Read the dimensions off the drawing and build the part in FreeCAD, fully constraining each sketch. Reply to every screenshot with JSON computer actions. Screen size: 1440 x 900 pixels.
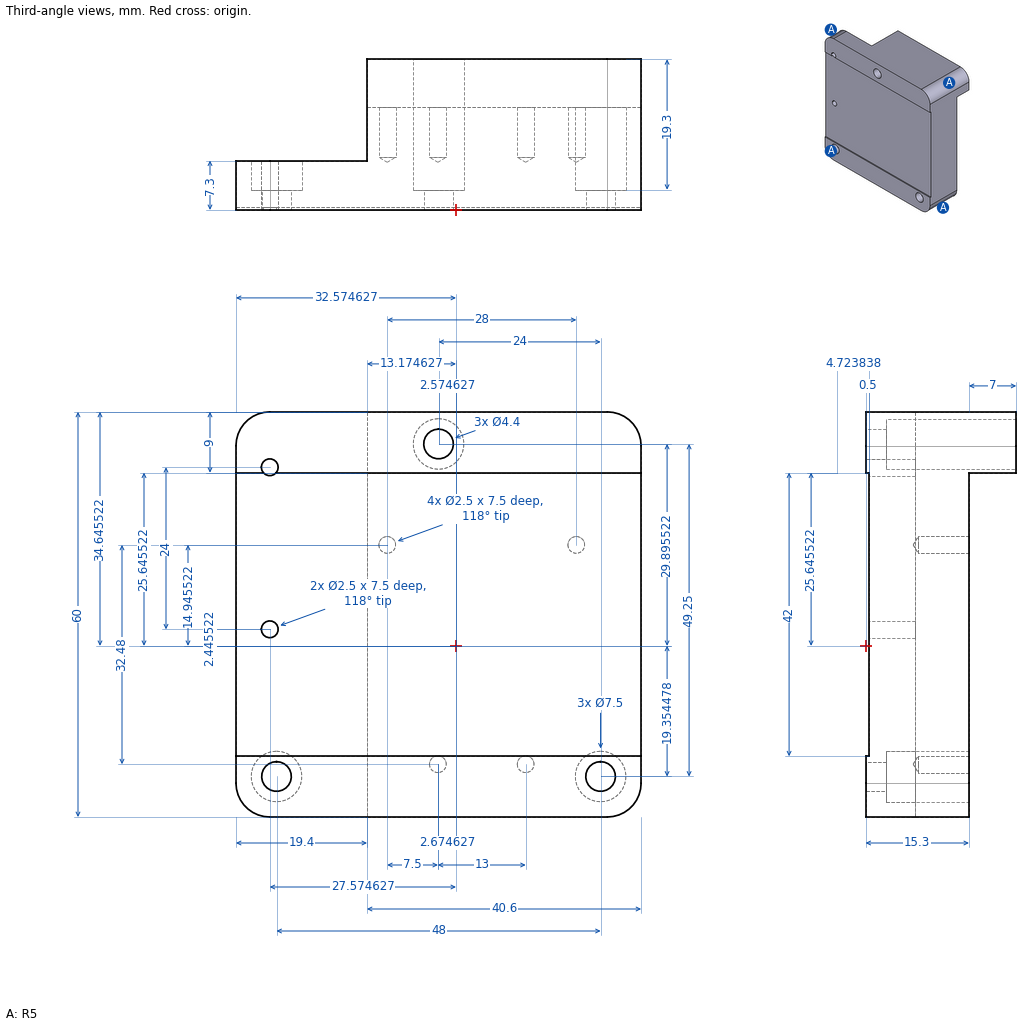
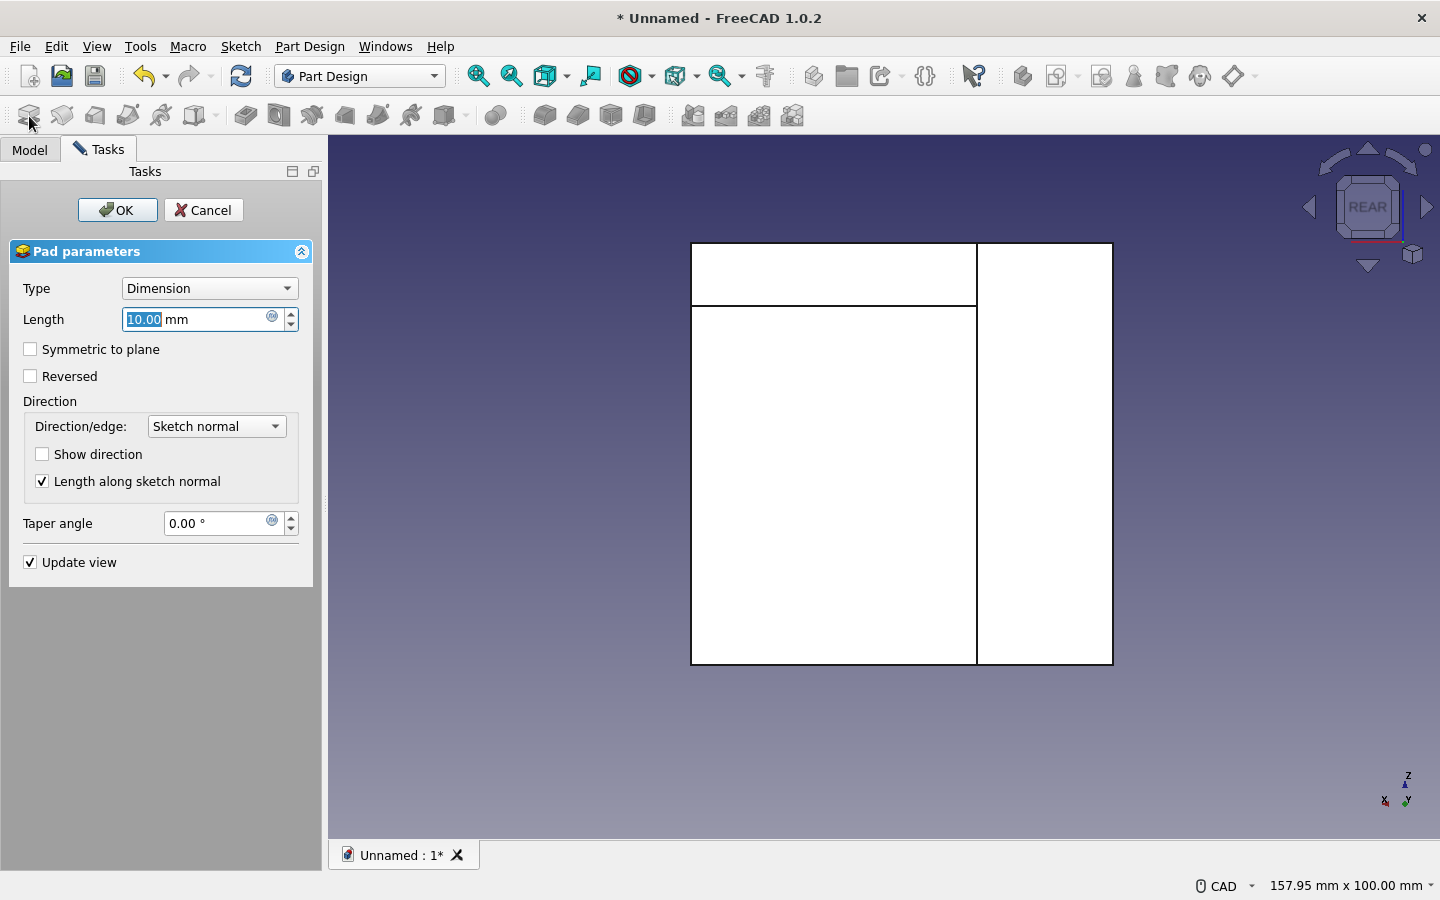
{"action": "type", "text": "7"}
{"action": "key", "text": "Tab"}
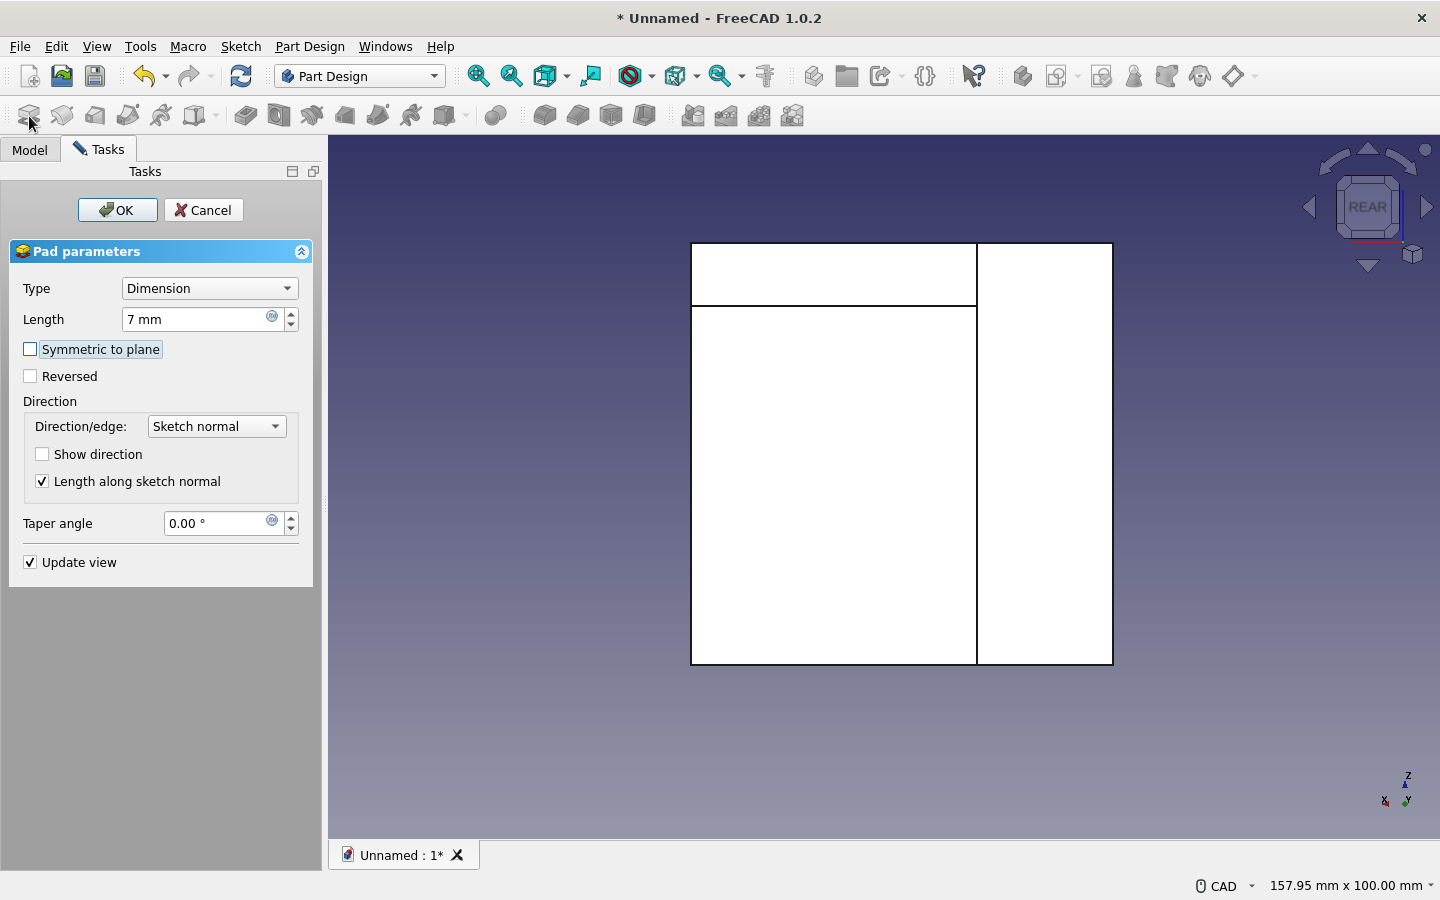
{"action": "left_click", "coordinate": [118, 210]}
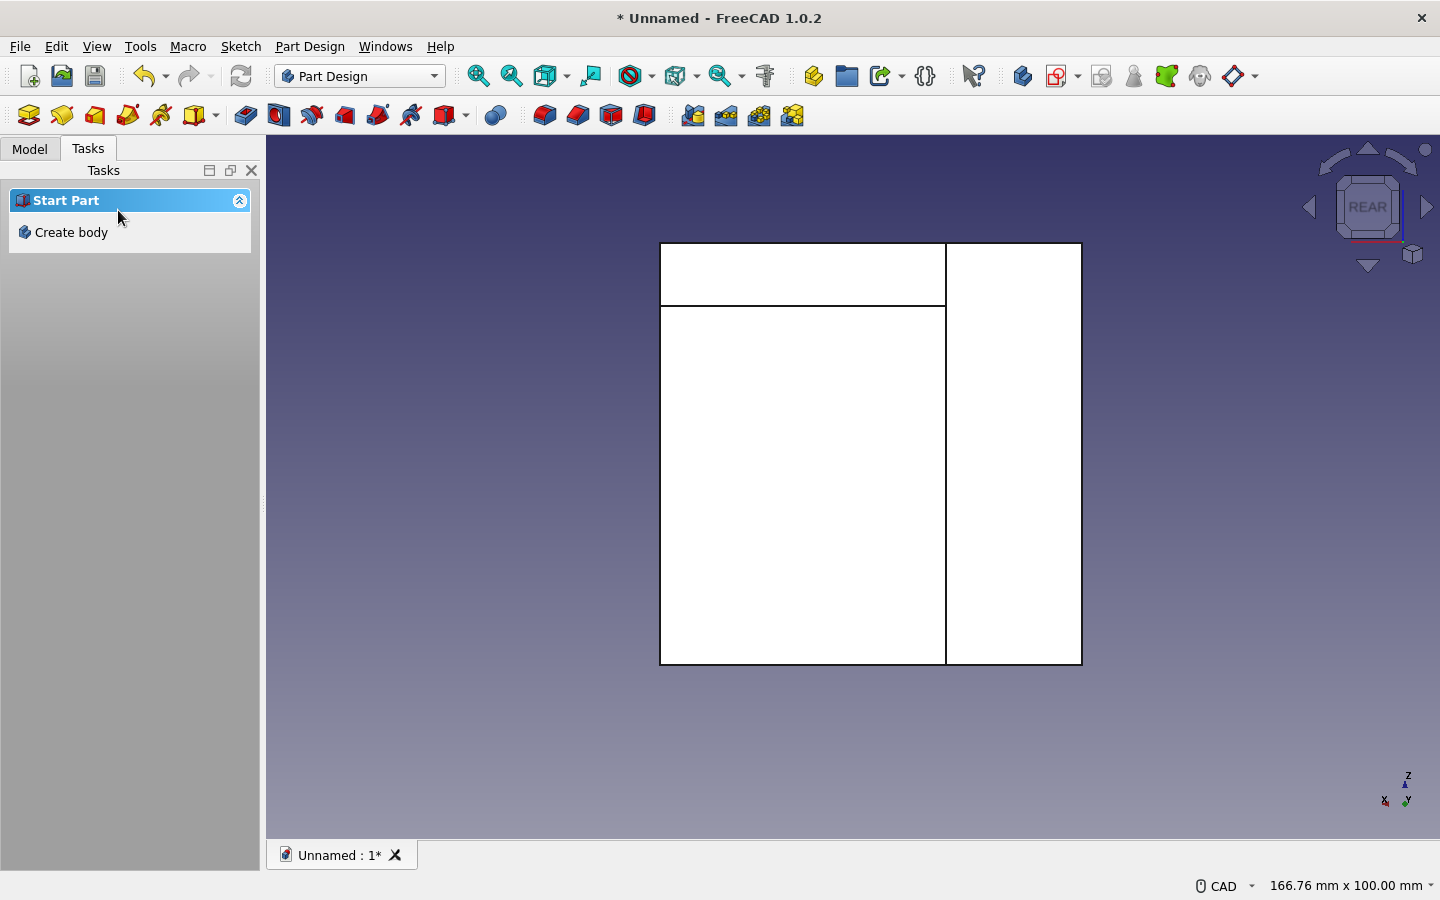
{"action": "left_click", "coordinate": [1014, 333]}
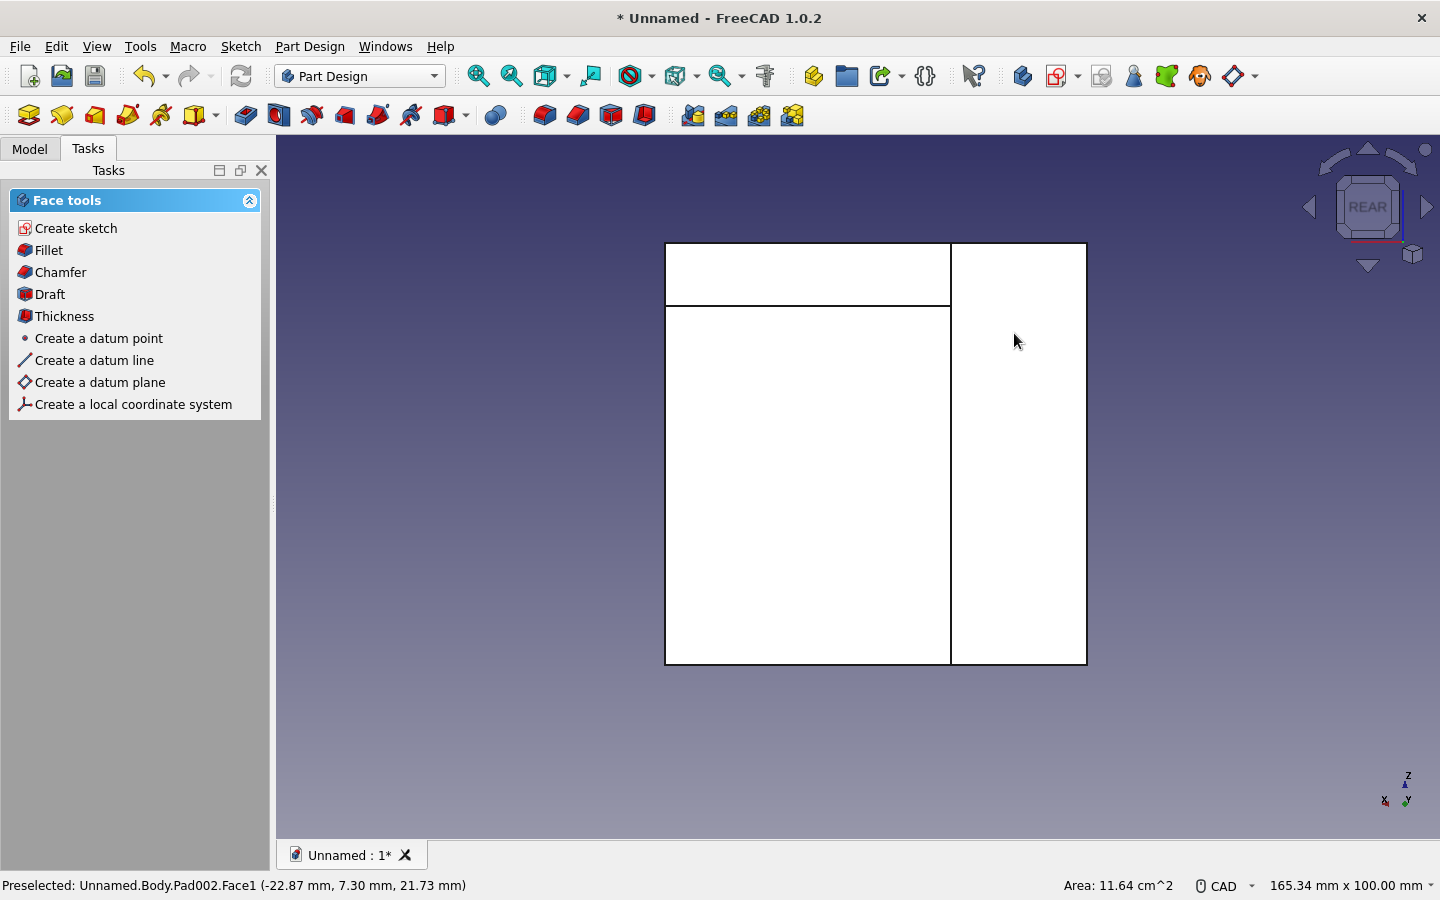
{"action": "left_click", "coordinate": [1056, 76]}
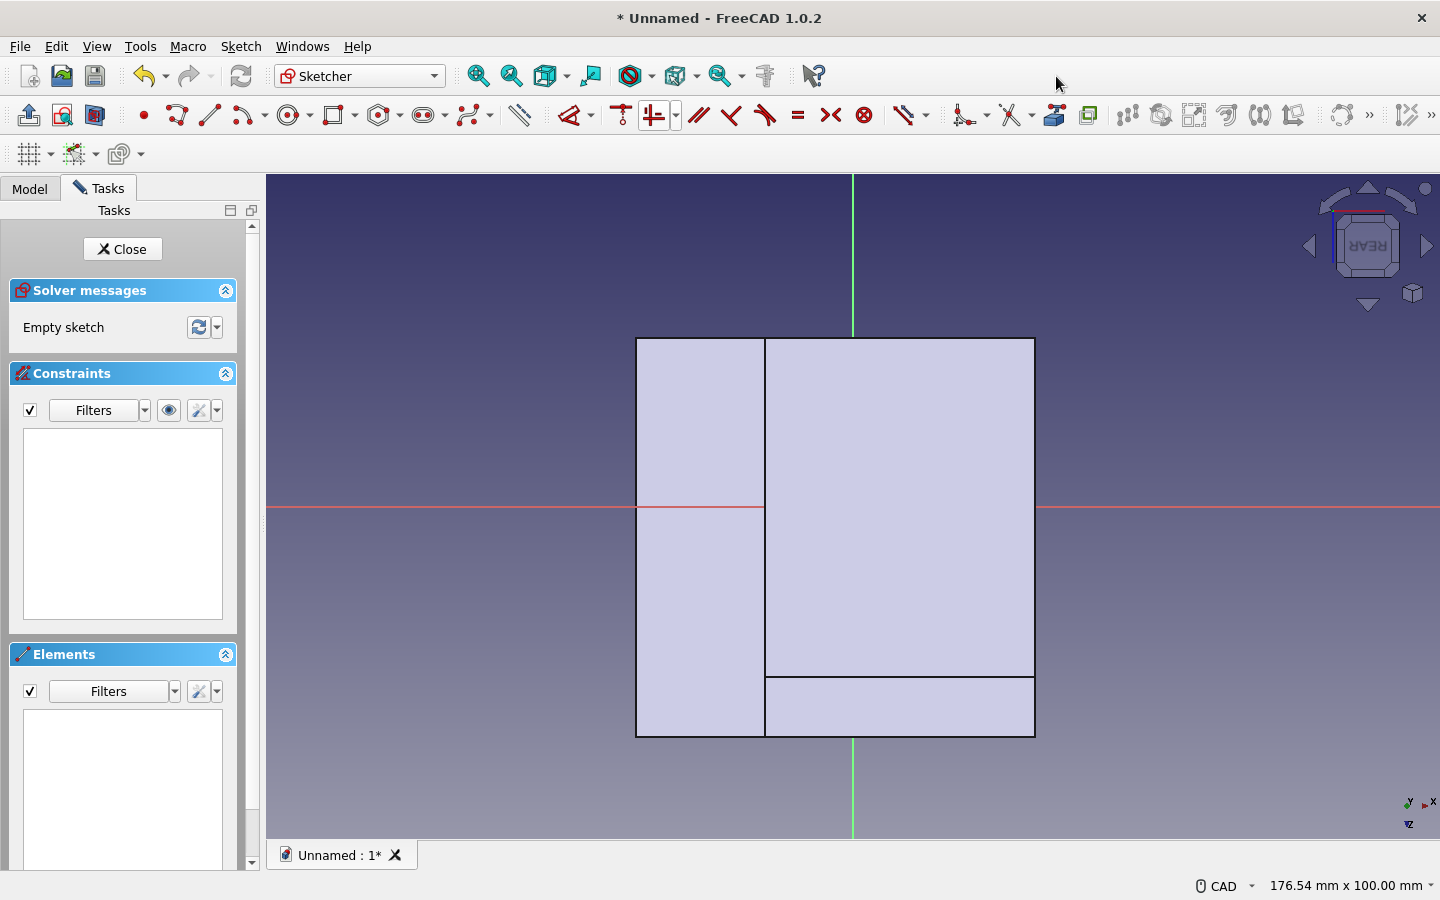
{"action": "scroll", "coordinate": [735, 674], "scroll_direction": "up", "scroll_amount": 4}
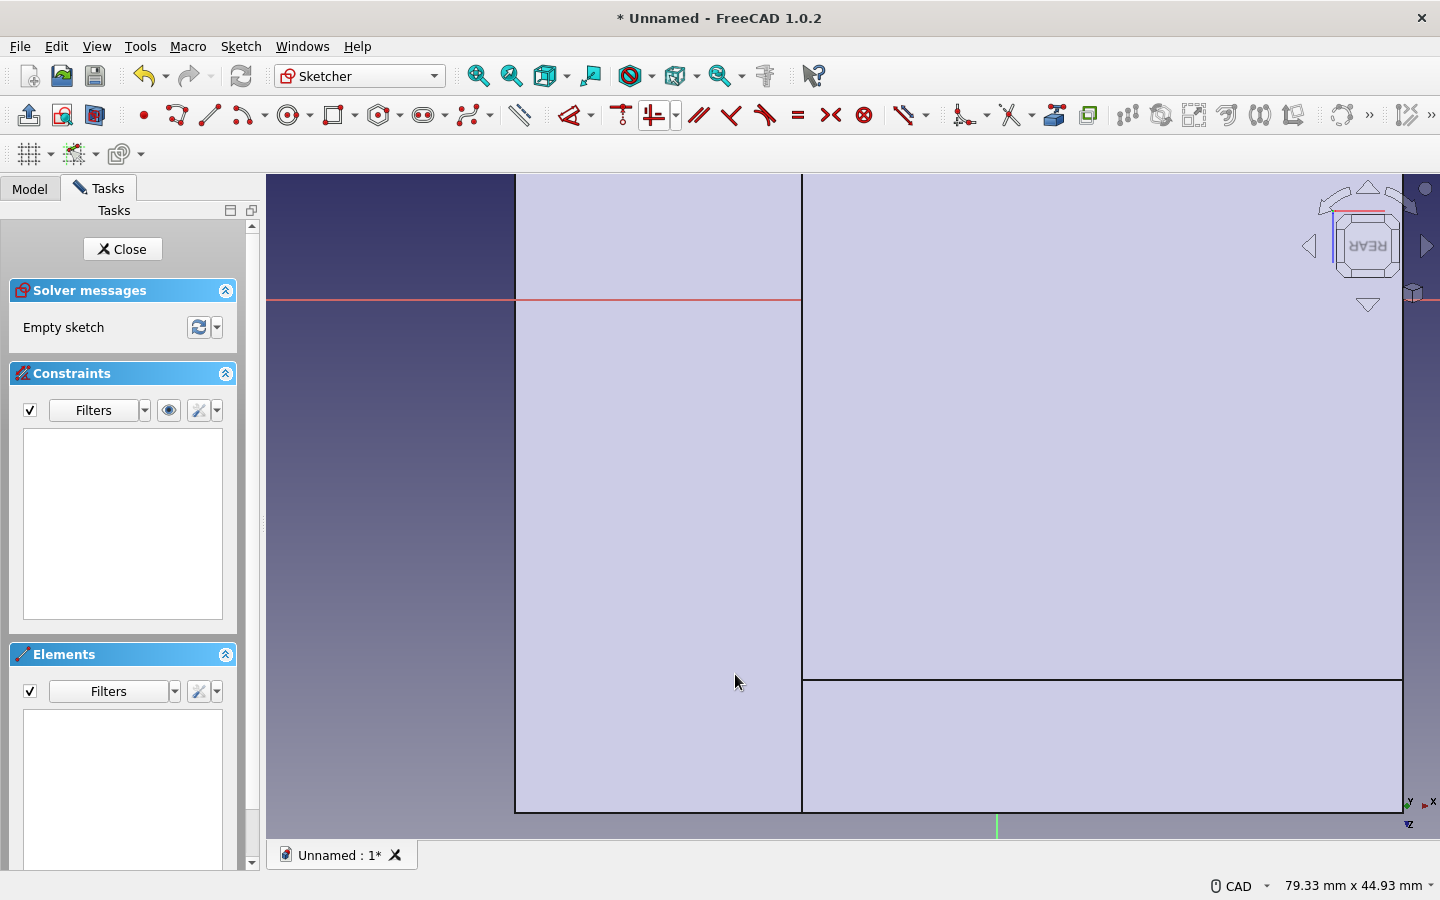
{"action": "left_click", "coordinate": [288, 116]}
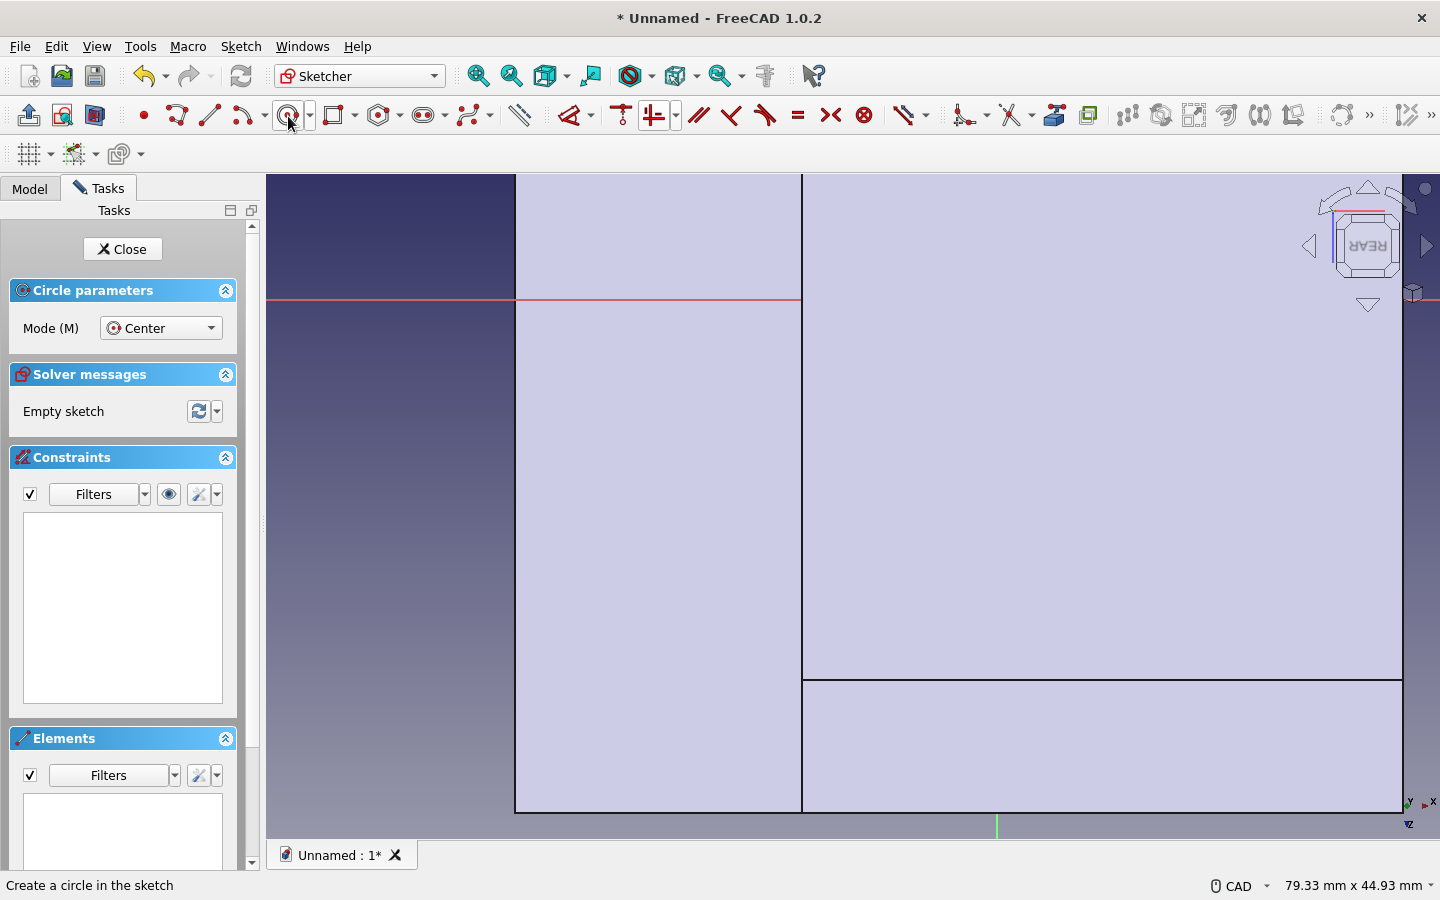
{"action": "scroll", "coordinate": [589, 336], "scroll_direction": "up", "scroll_amount": 2}